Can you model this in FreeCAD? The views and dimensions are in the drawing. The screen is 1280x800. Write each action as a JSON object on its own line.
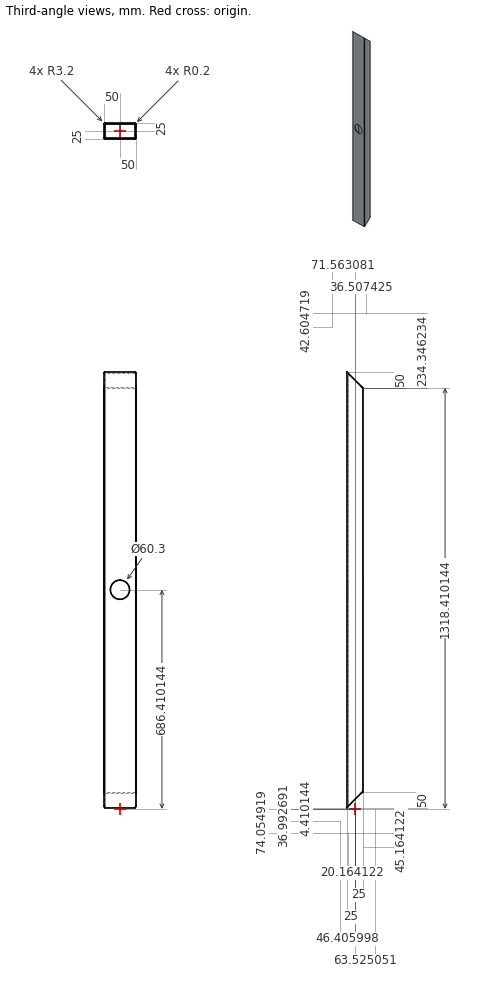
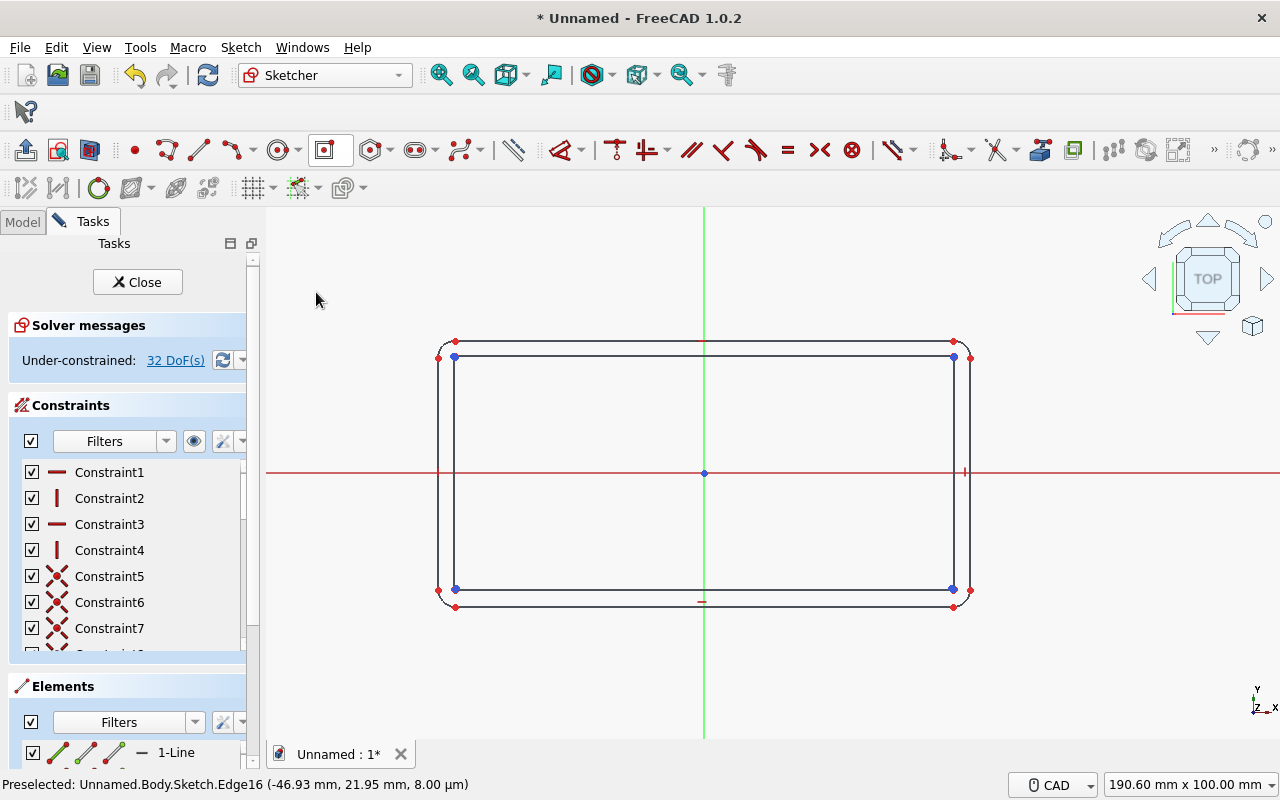
{"action": "left_click", "coordinate": [804, 341]}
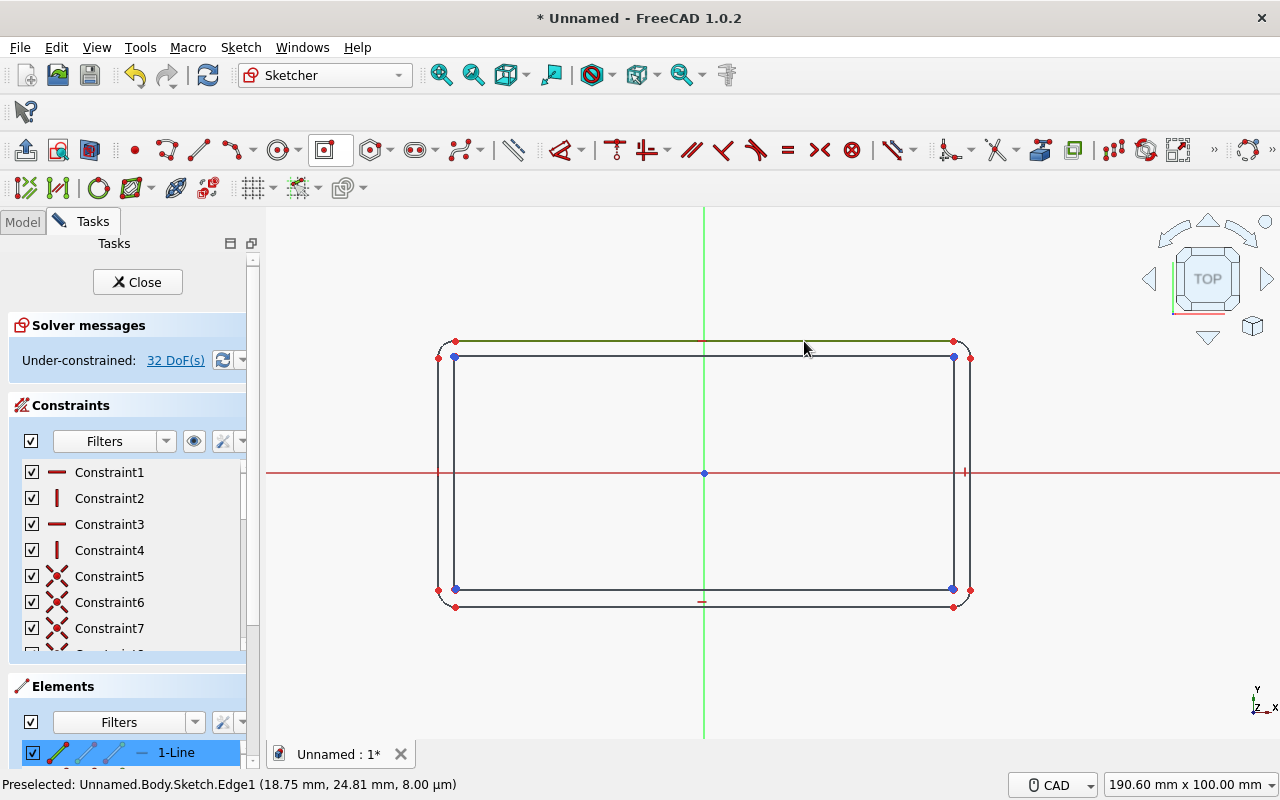
{"action": "left_click", "coordinate": [443, 346]}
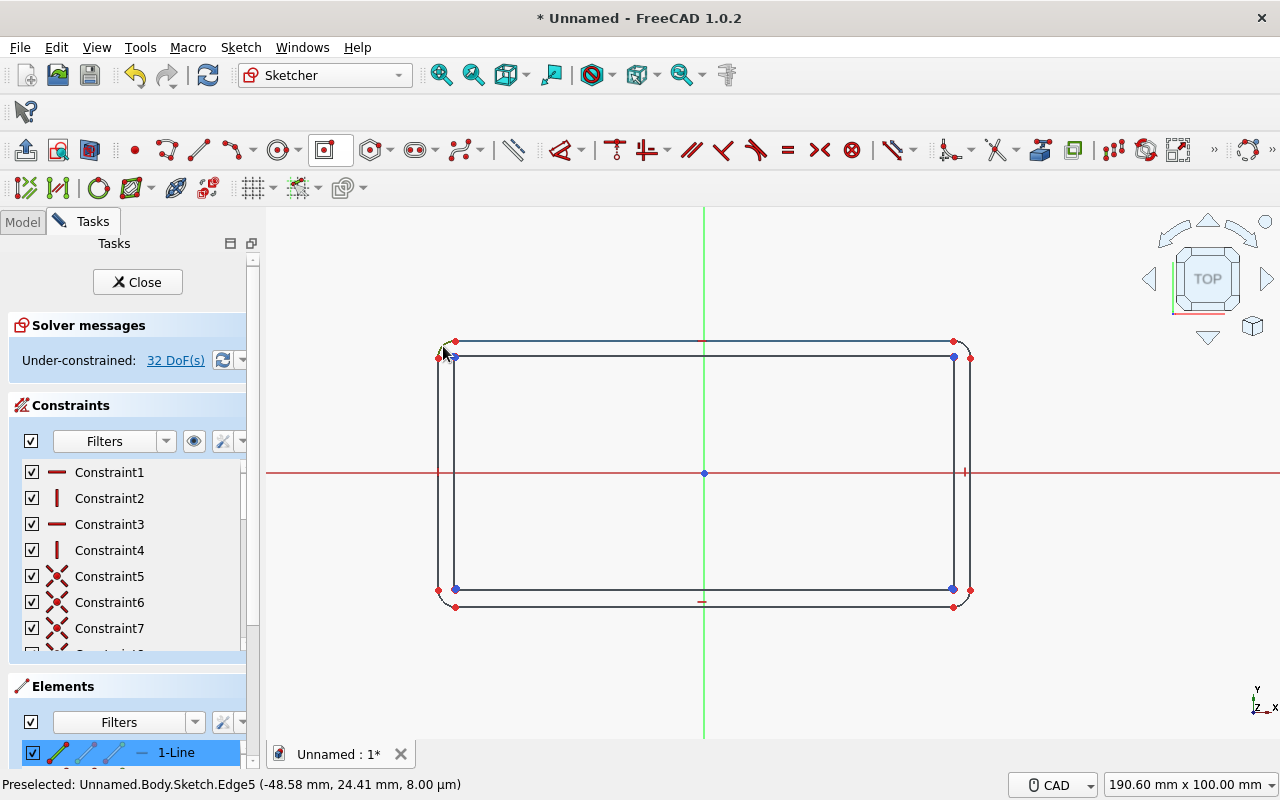
{"action": "left_click", "coordinate": [756, 150]}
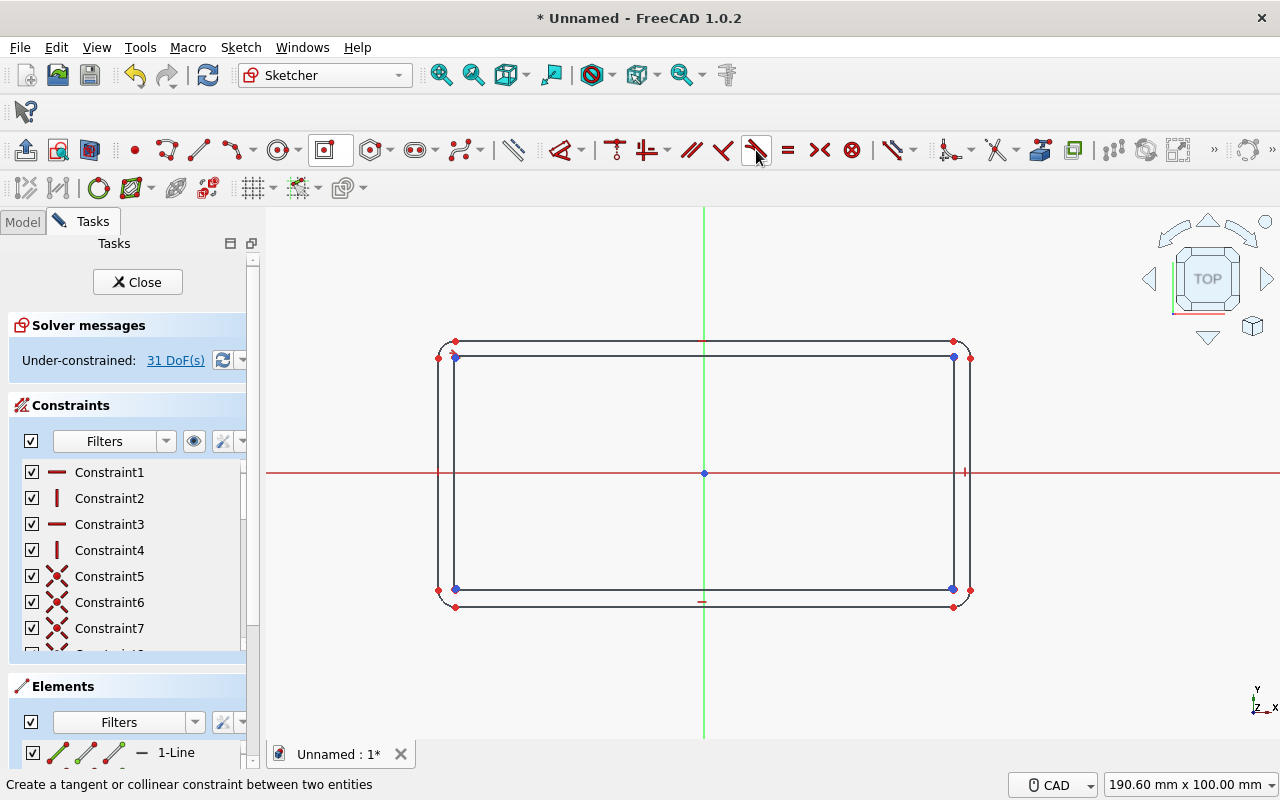
{"action": "left_click", "coordinate": [804, 341]}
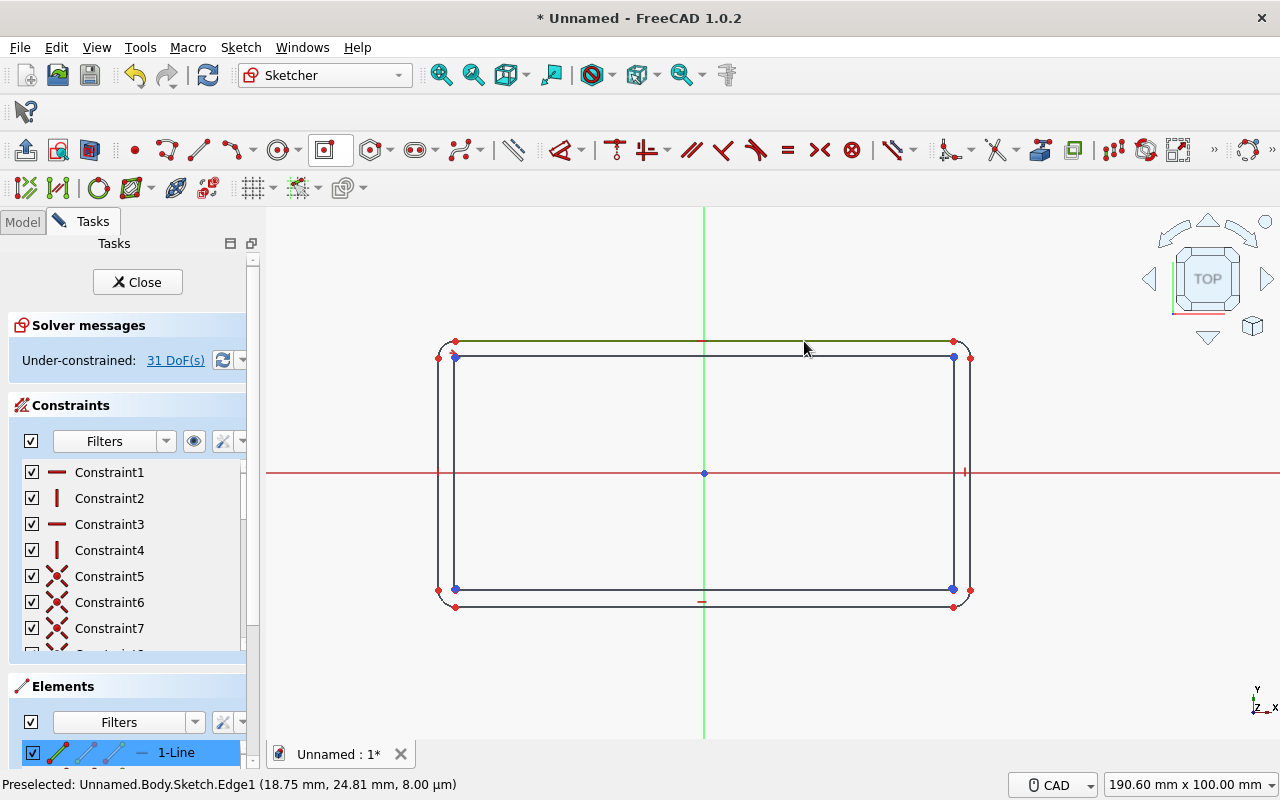
{"action": "left_click", "coordinate": [966, 346]}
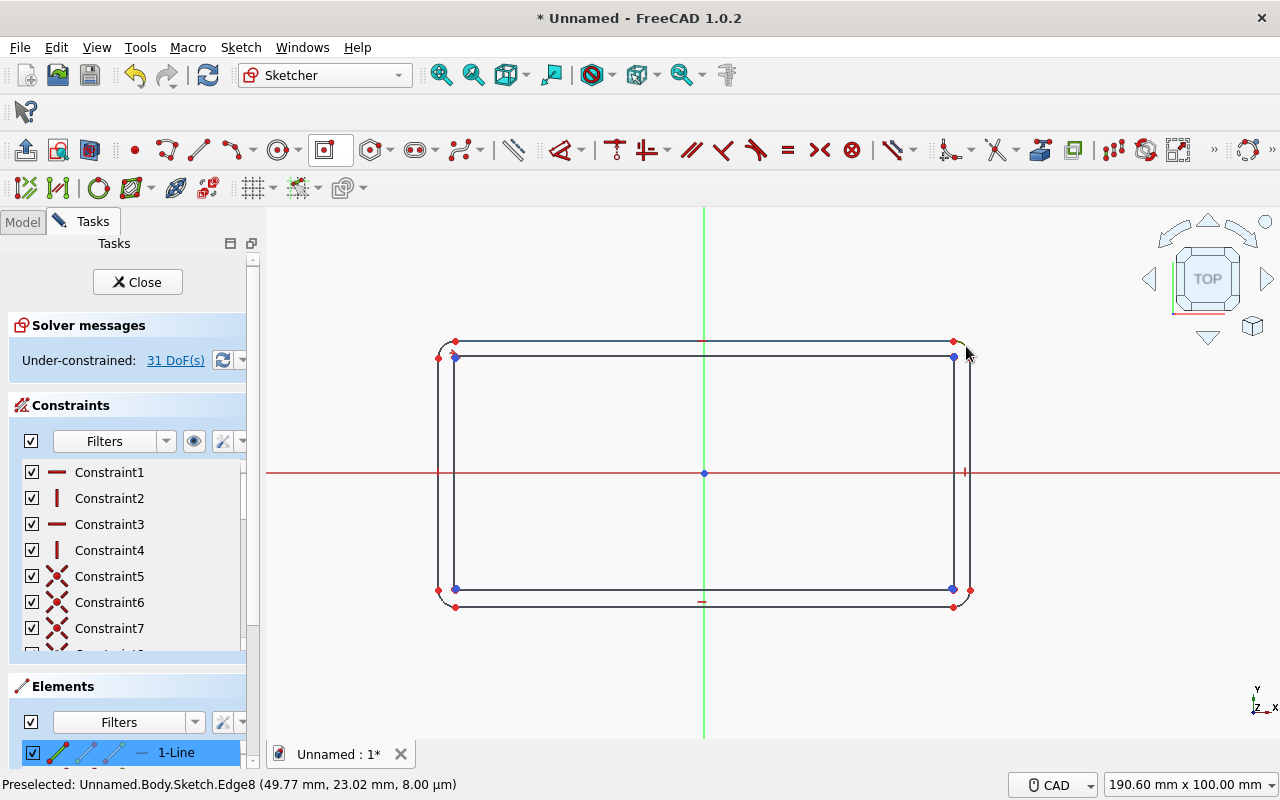
{"action": "left_click", "coordinate": [756, 150]}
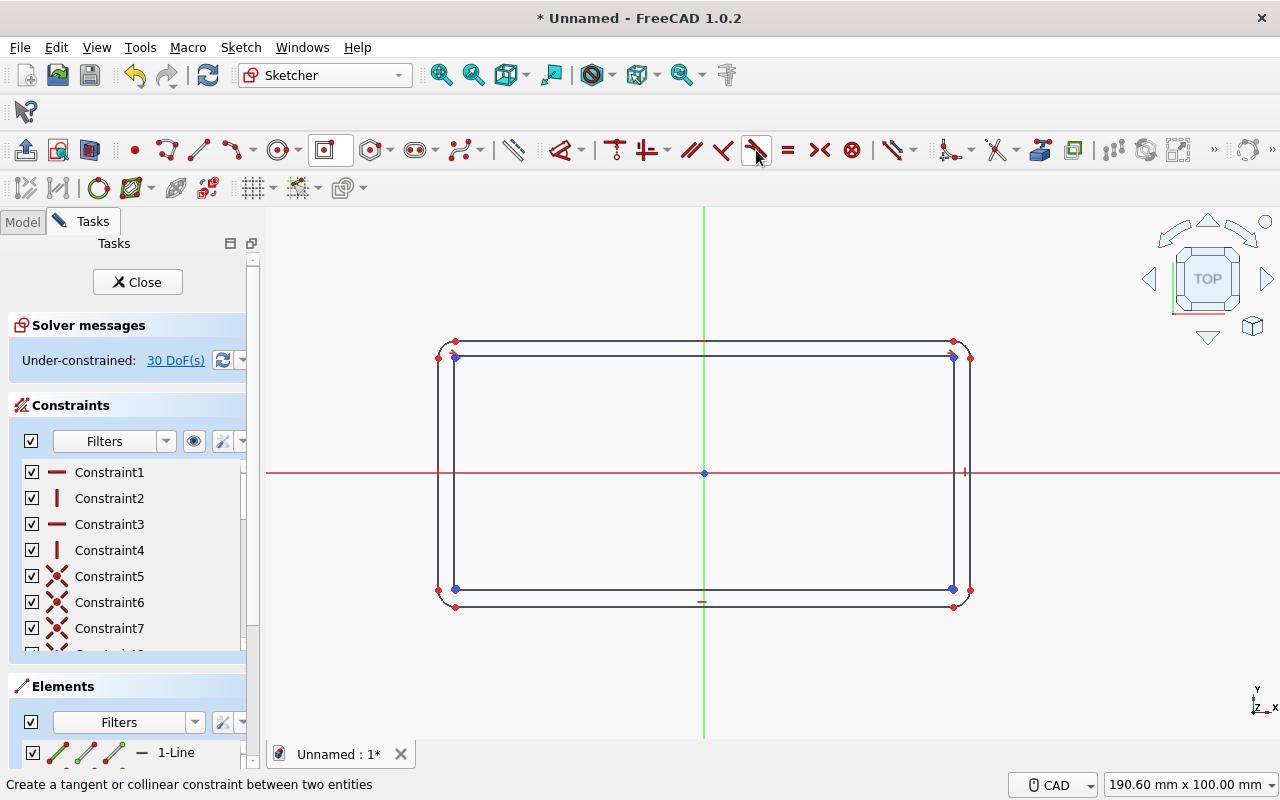
{"action": "left_click", "coordinate": [438, 428]}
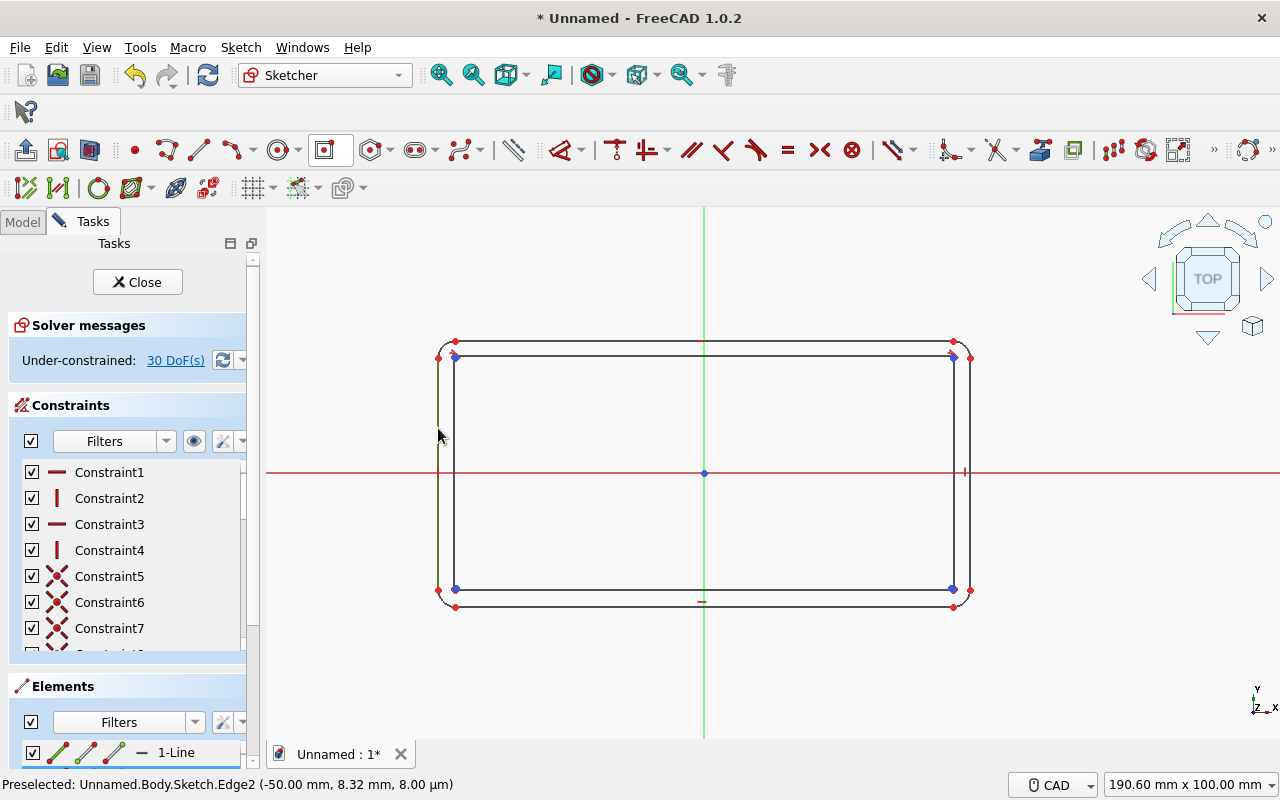
{"action": "left_click", "coordinate": [443, 346]}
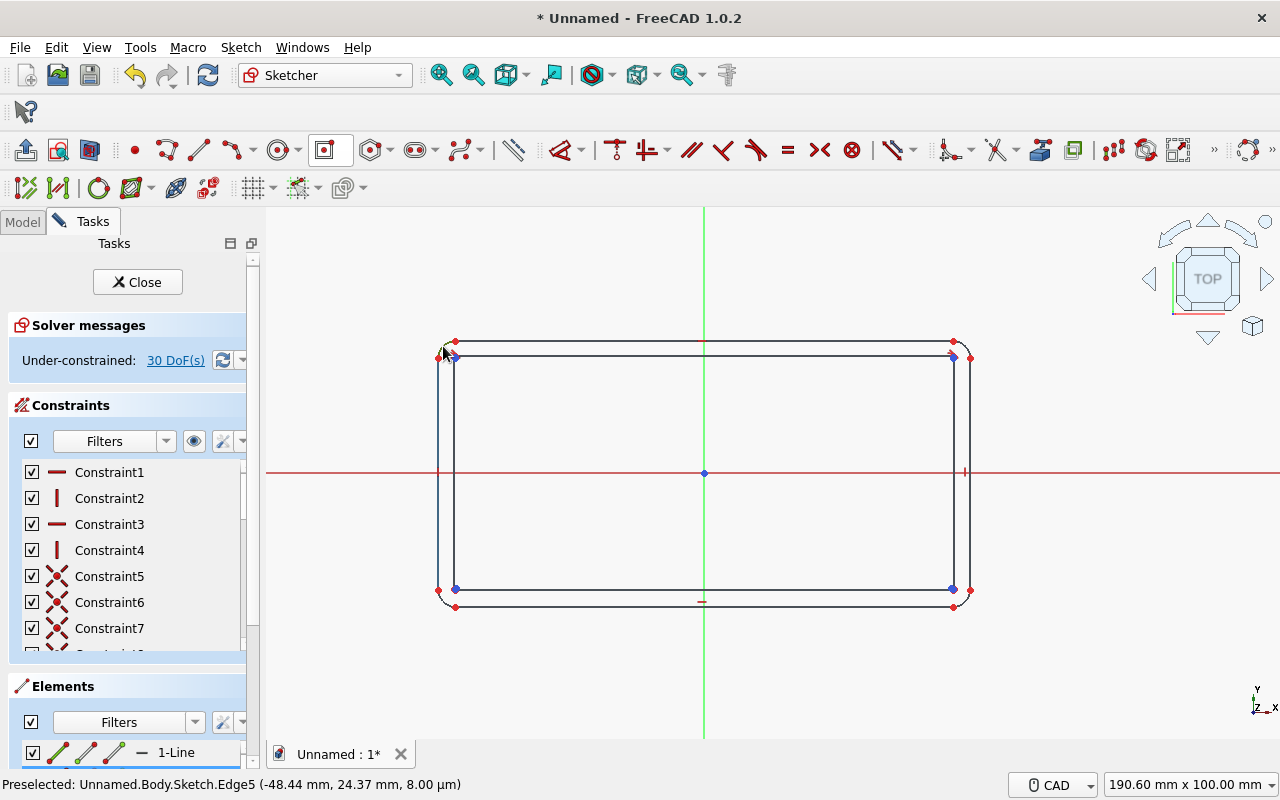
{"action": "left_click", "coordinate": [756, 150]}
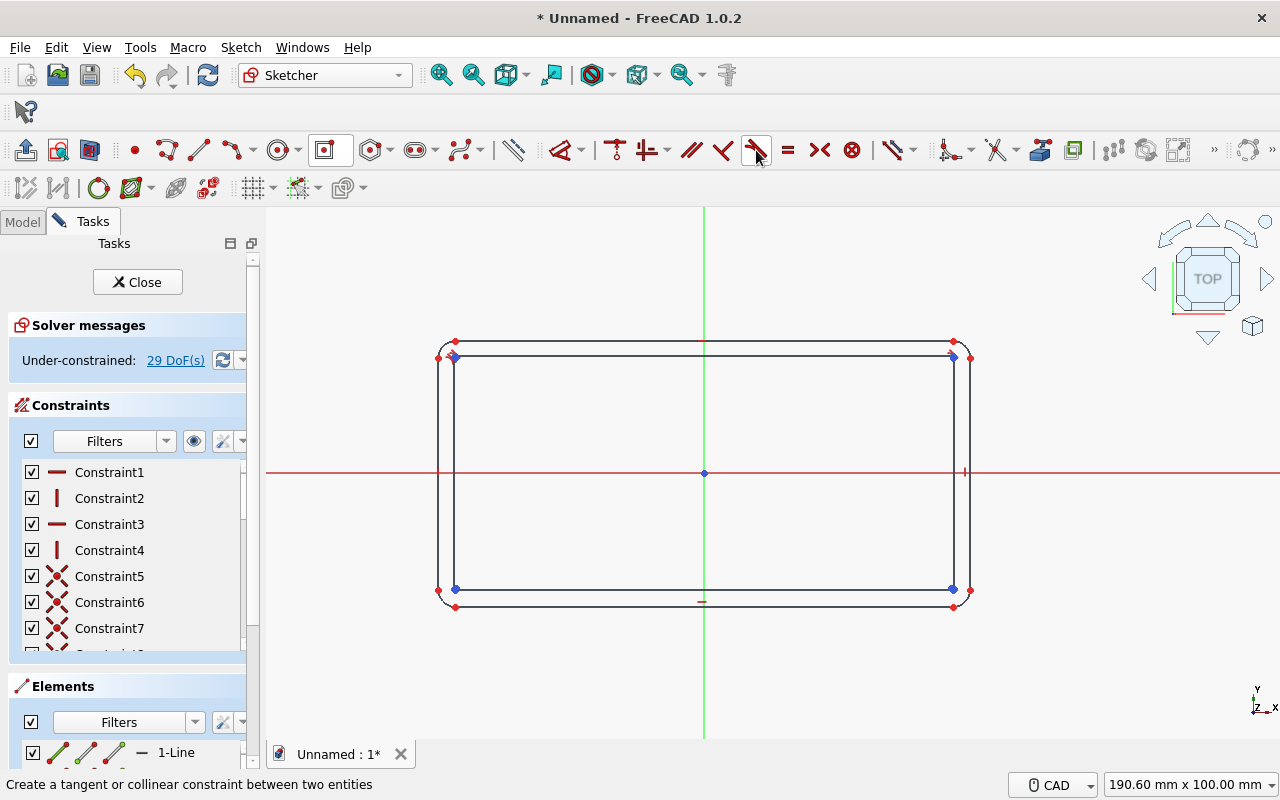
{"action": "left_click", "coordinate": [438, 428]}